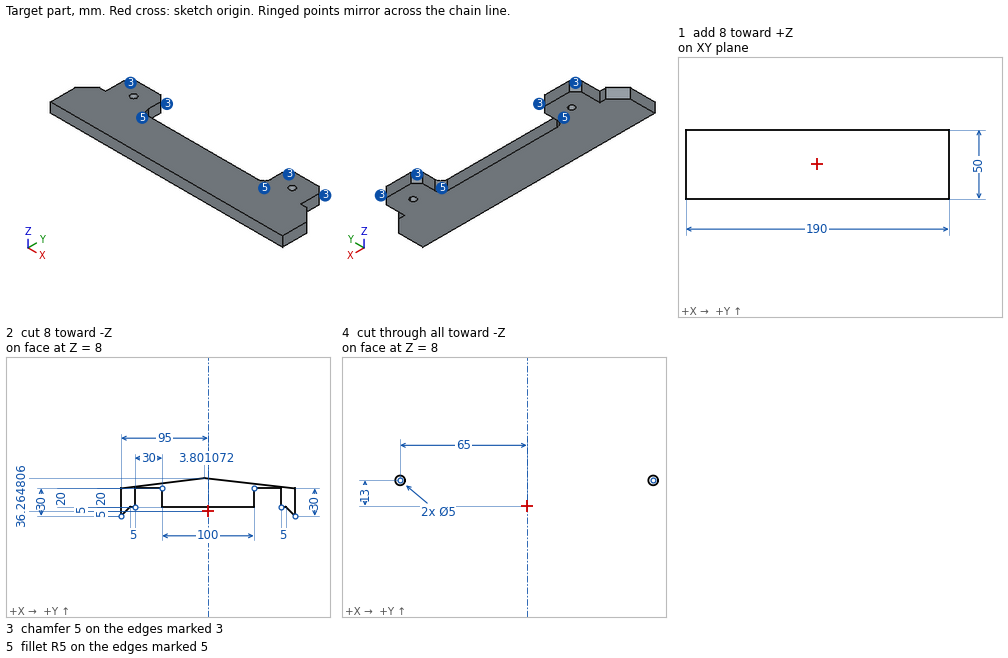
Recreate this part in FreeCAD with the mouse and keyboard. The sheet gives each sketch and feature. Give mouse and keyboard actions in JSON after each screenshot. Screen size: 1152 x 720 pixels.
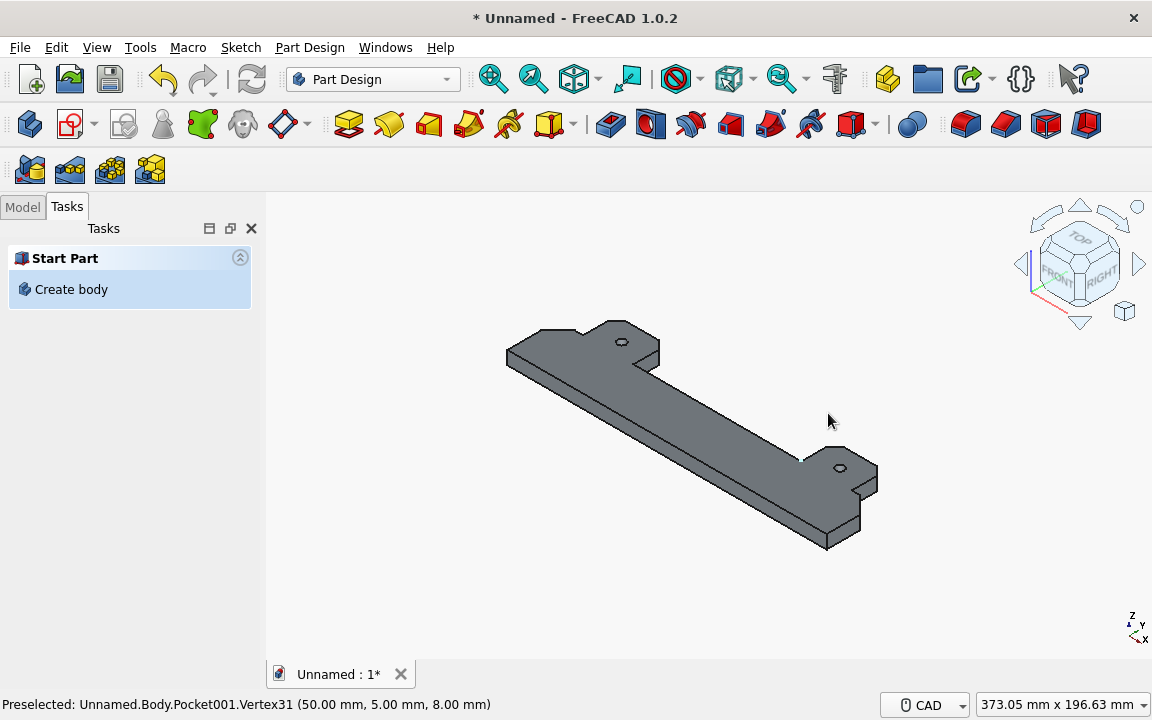
{"action": "scroll", "coordinate": [801, 468], "scroll_direction": "up", "scroll_amount": 4}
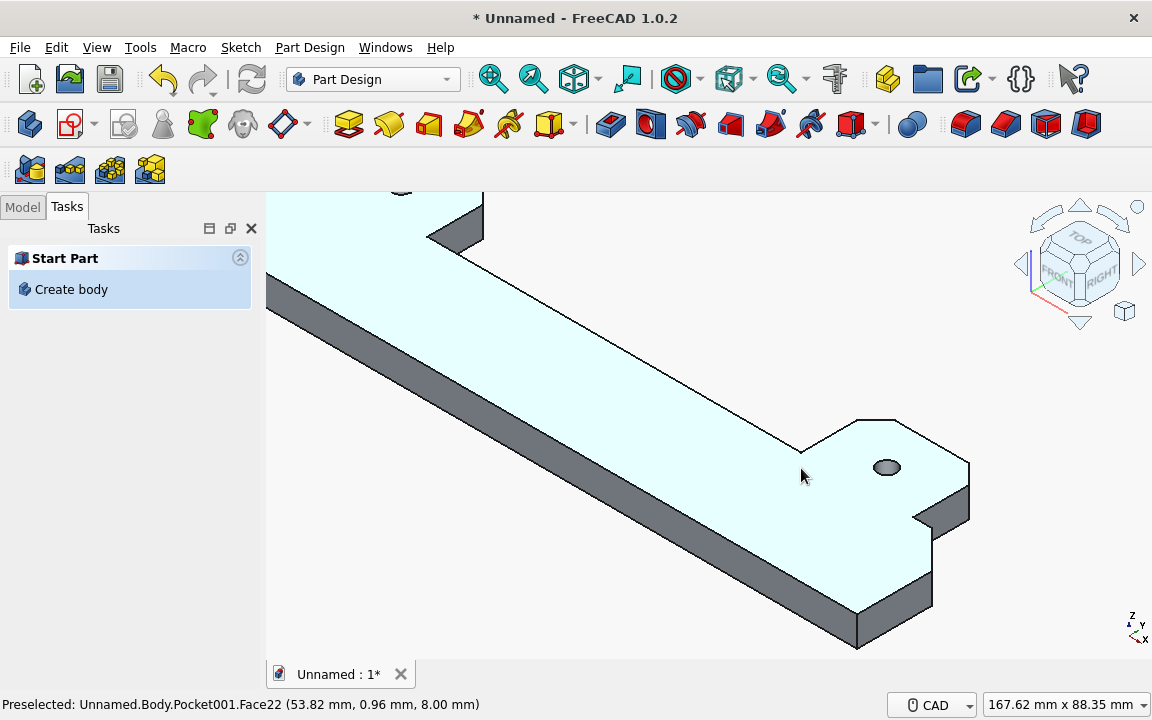
{"action": "left_click", "coordinate": [494, 80]}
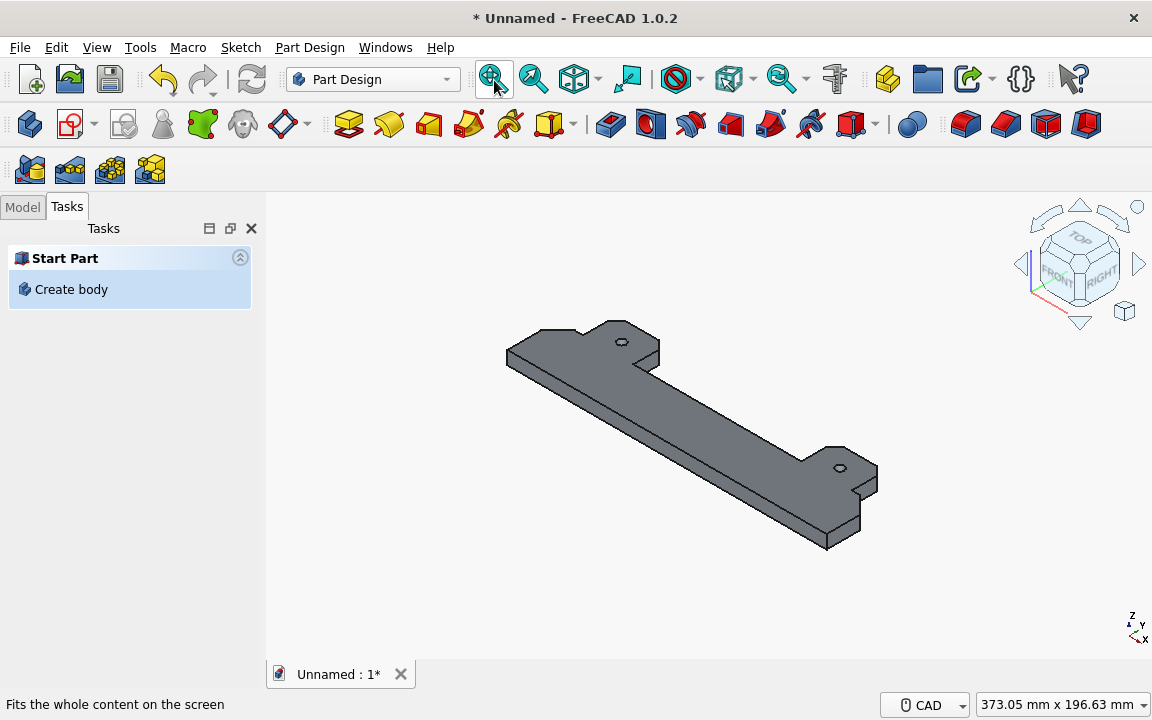
{"action": "key", "text": "1"}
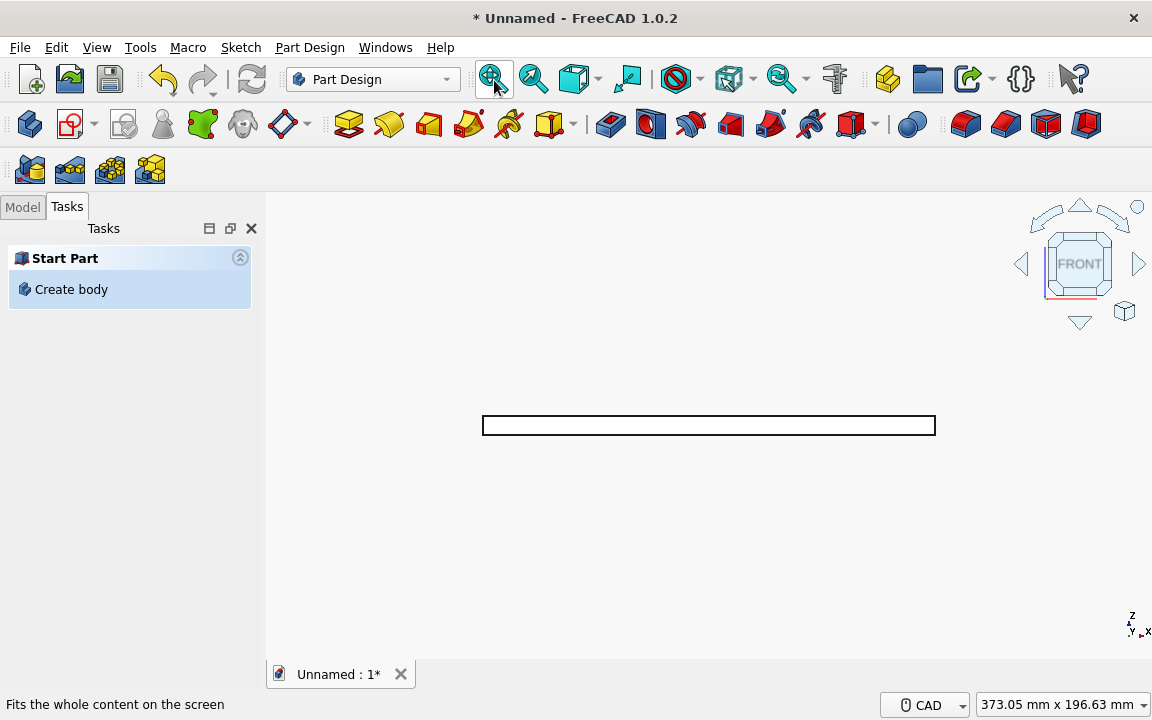
{"action": "scroll", "coordinate": [828, 424], "scroll_direction": "up", "scroll_amount": 4}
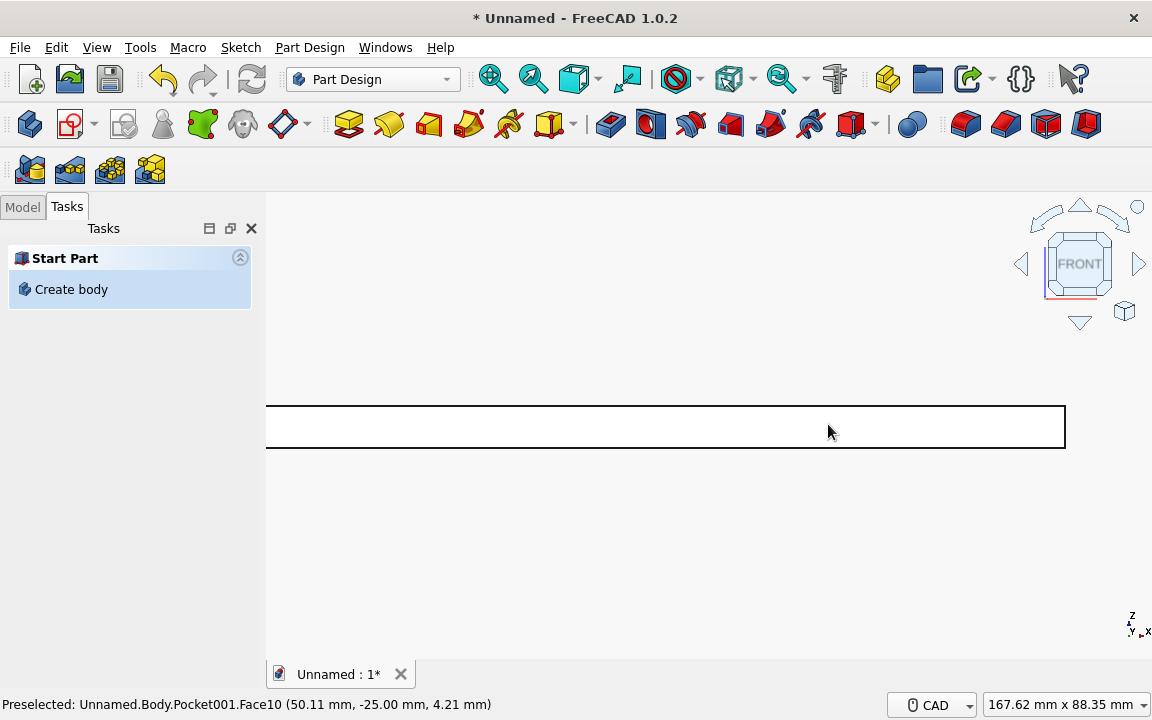
{"action": "left_click", "coordinate": [494, 80]}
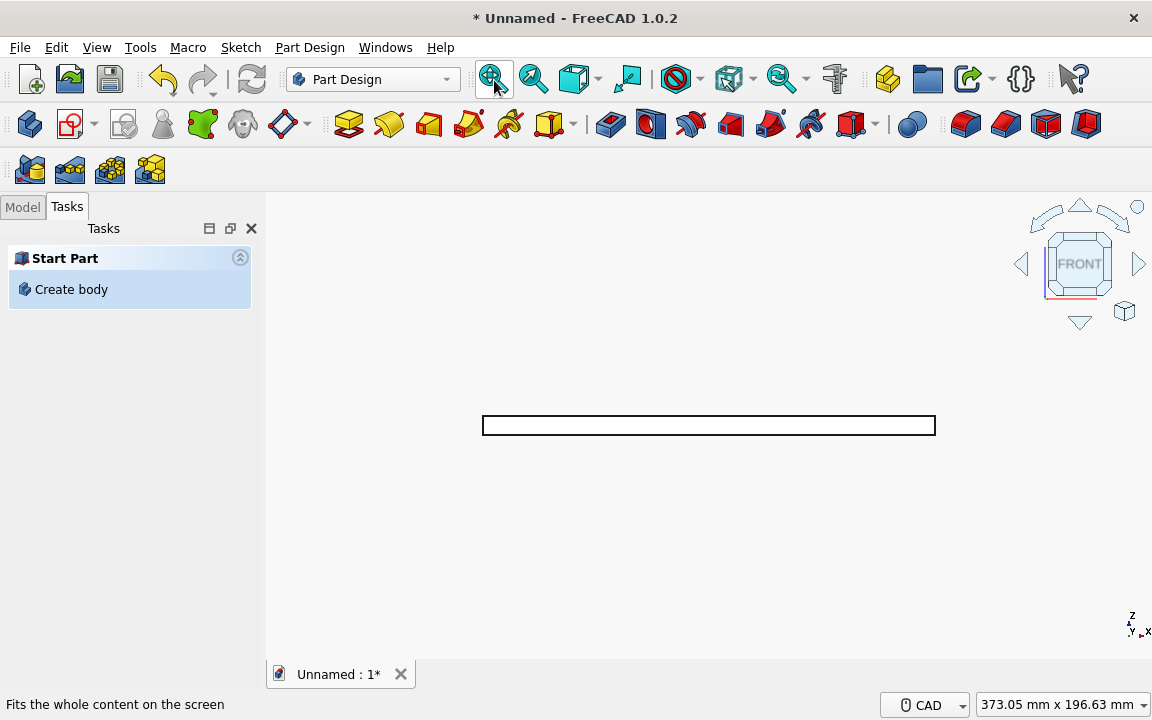
{"action": "key", "text": "3"}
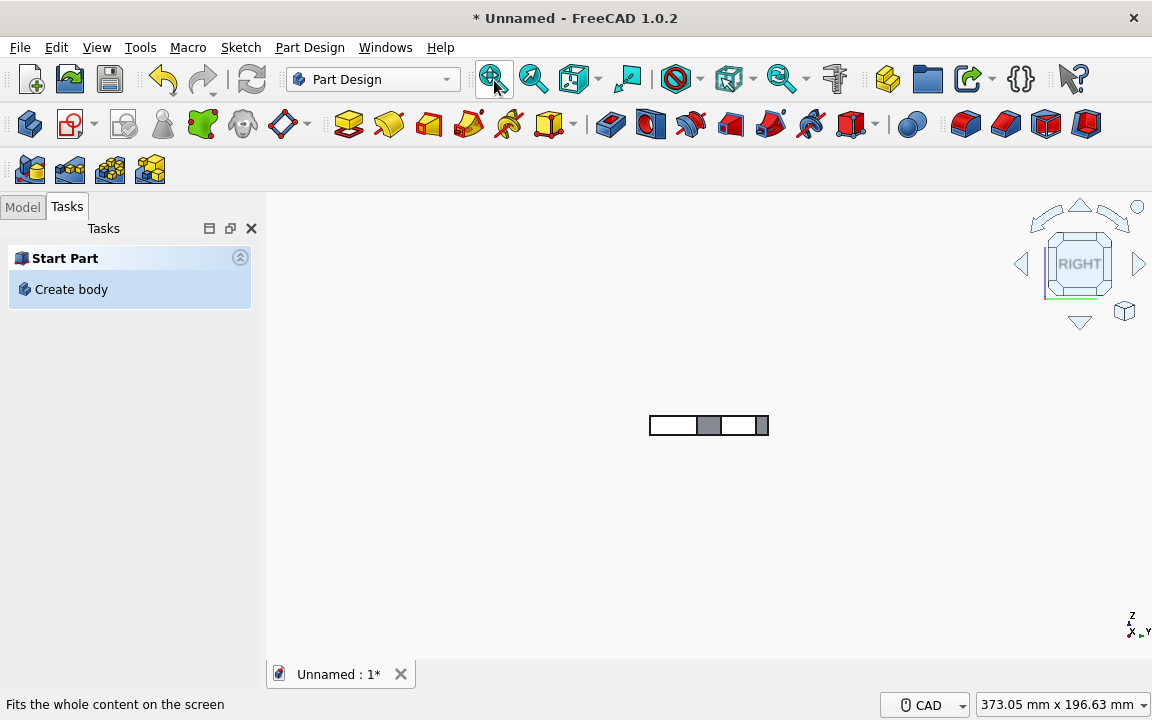
{"action": "left_click", "coordinate": [494, 80]}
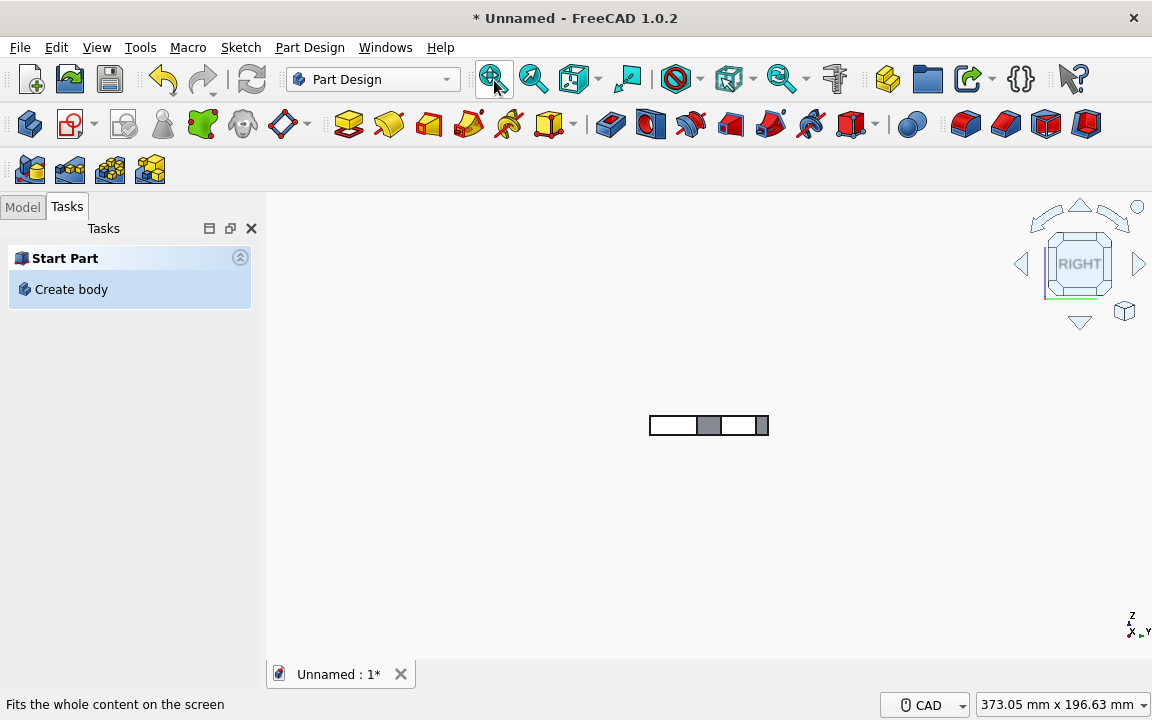
{"action": "scroll", "coordinate": [721, 424], "scroll_direction": "up", "scroll_amount": 4}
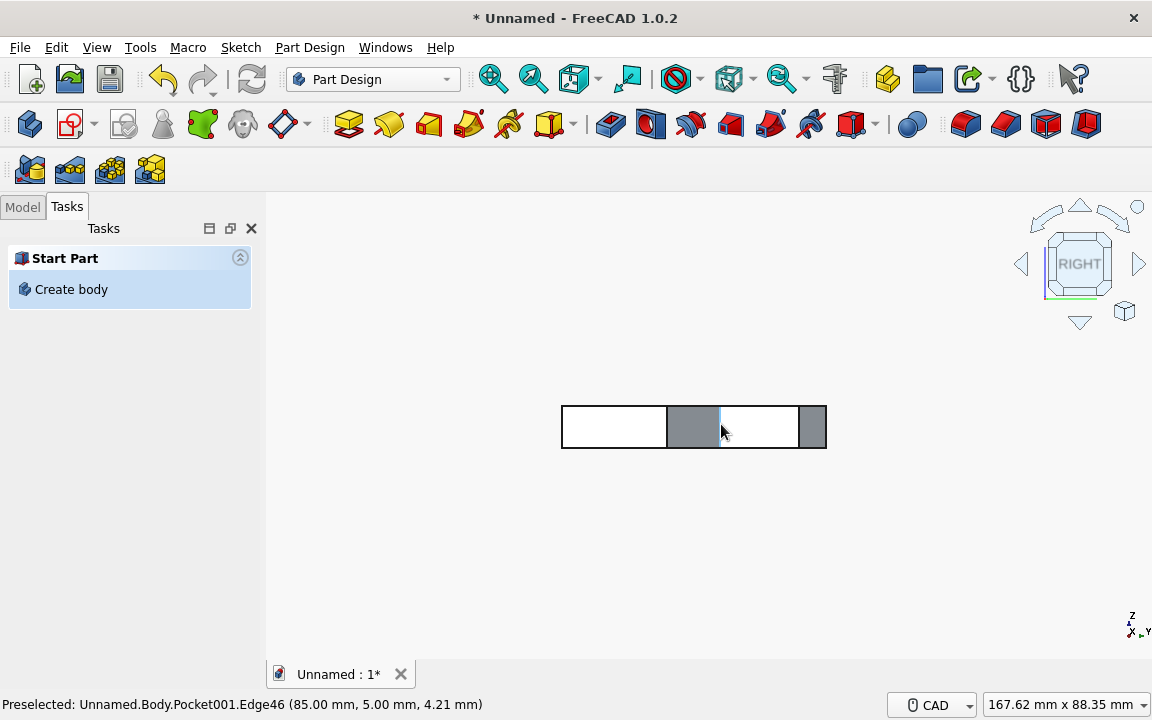
{"action": "key", "text": "v f"}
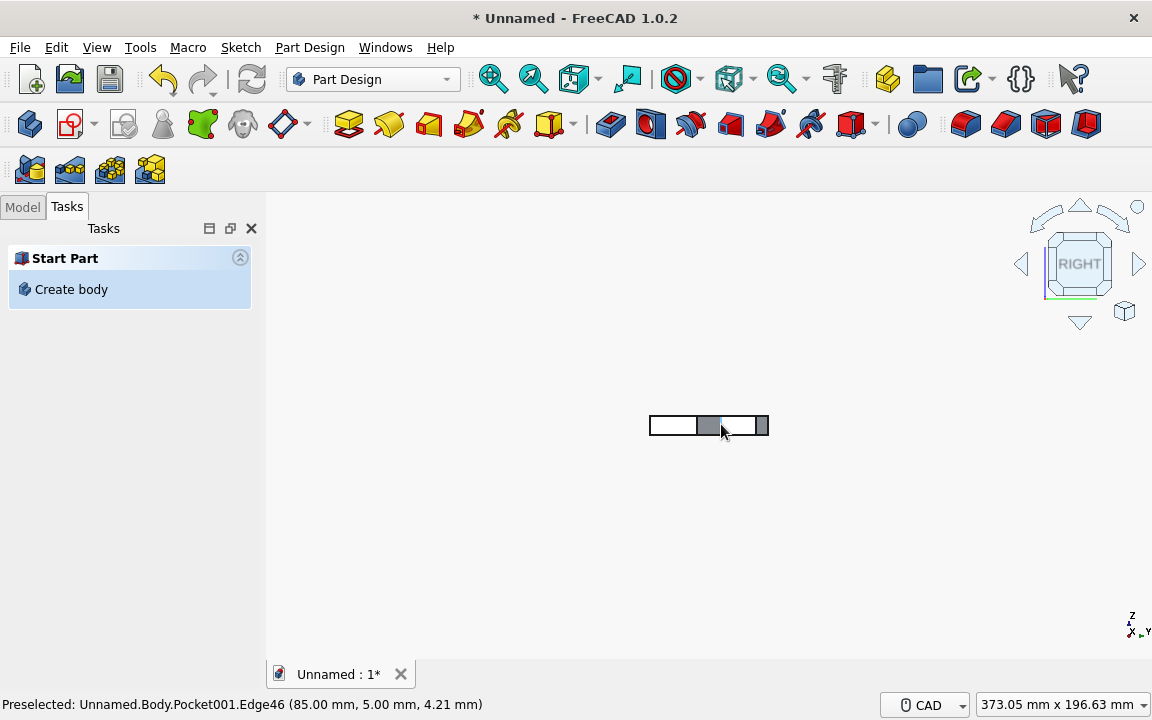
{"action": "key", "text": "5"}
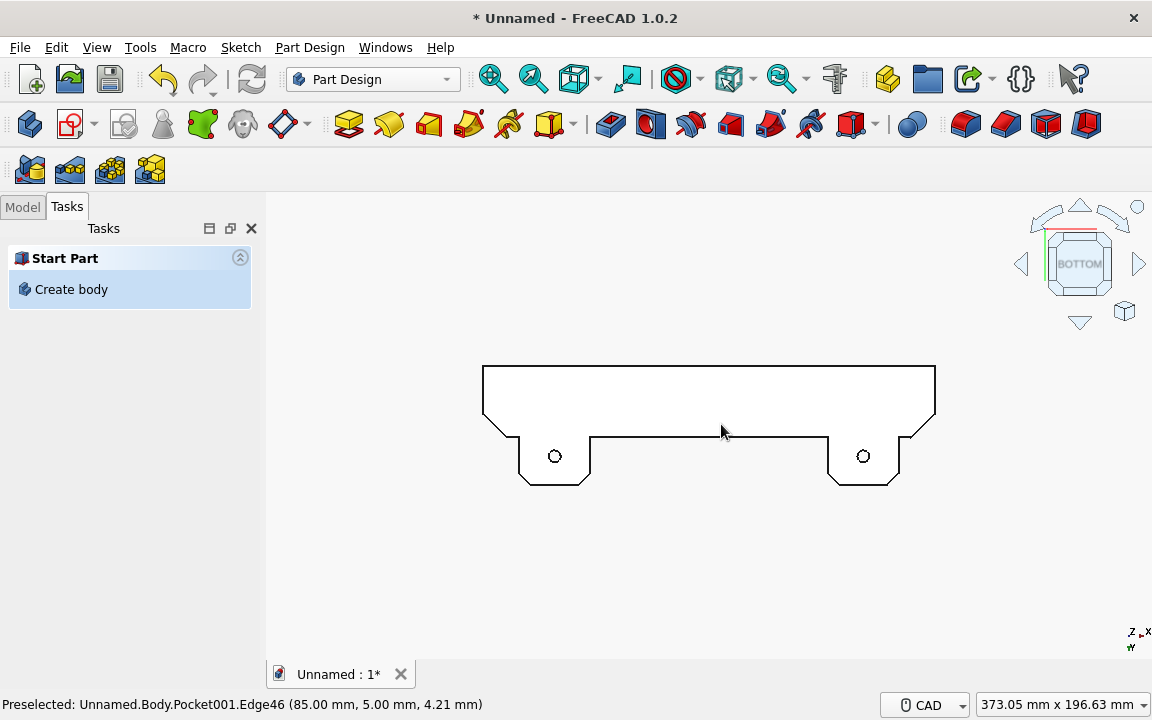
{"action": "scroll", "coordinate": [828, 436], "scroll_direction": "up", "scroll_amount": 4}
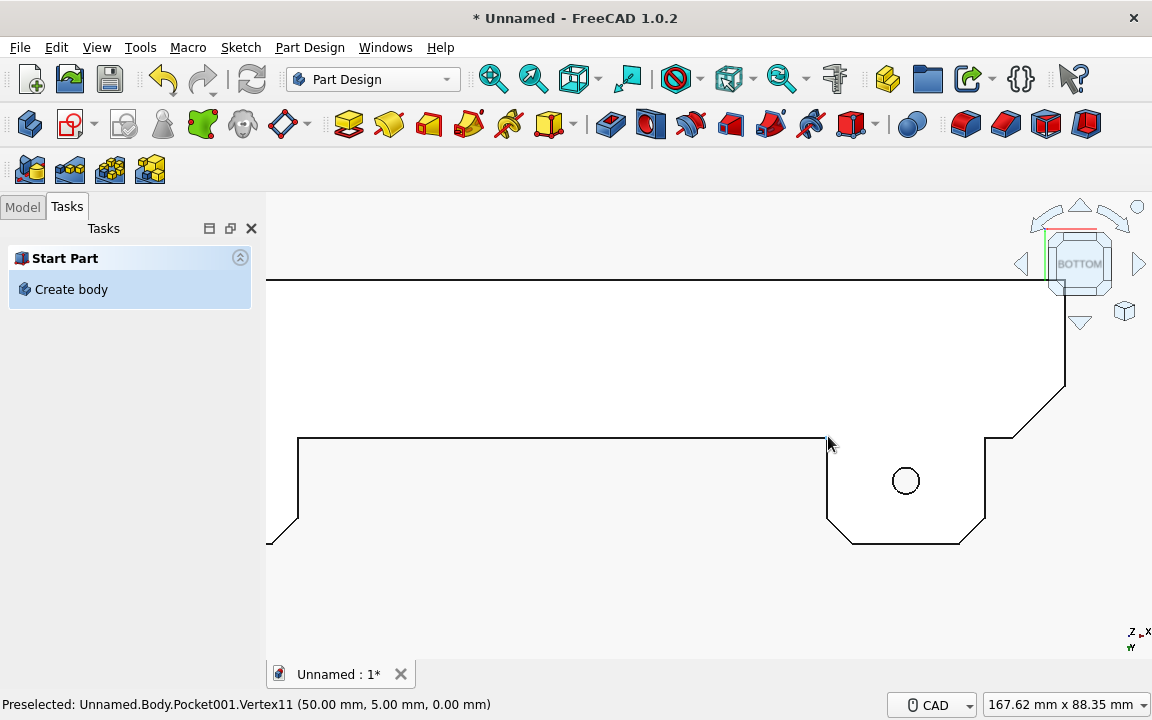
{"action": "left_click", "coordinate": [494, 80]}